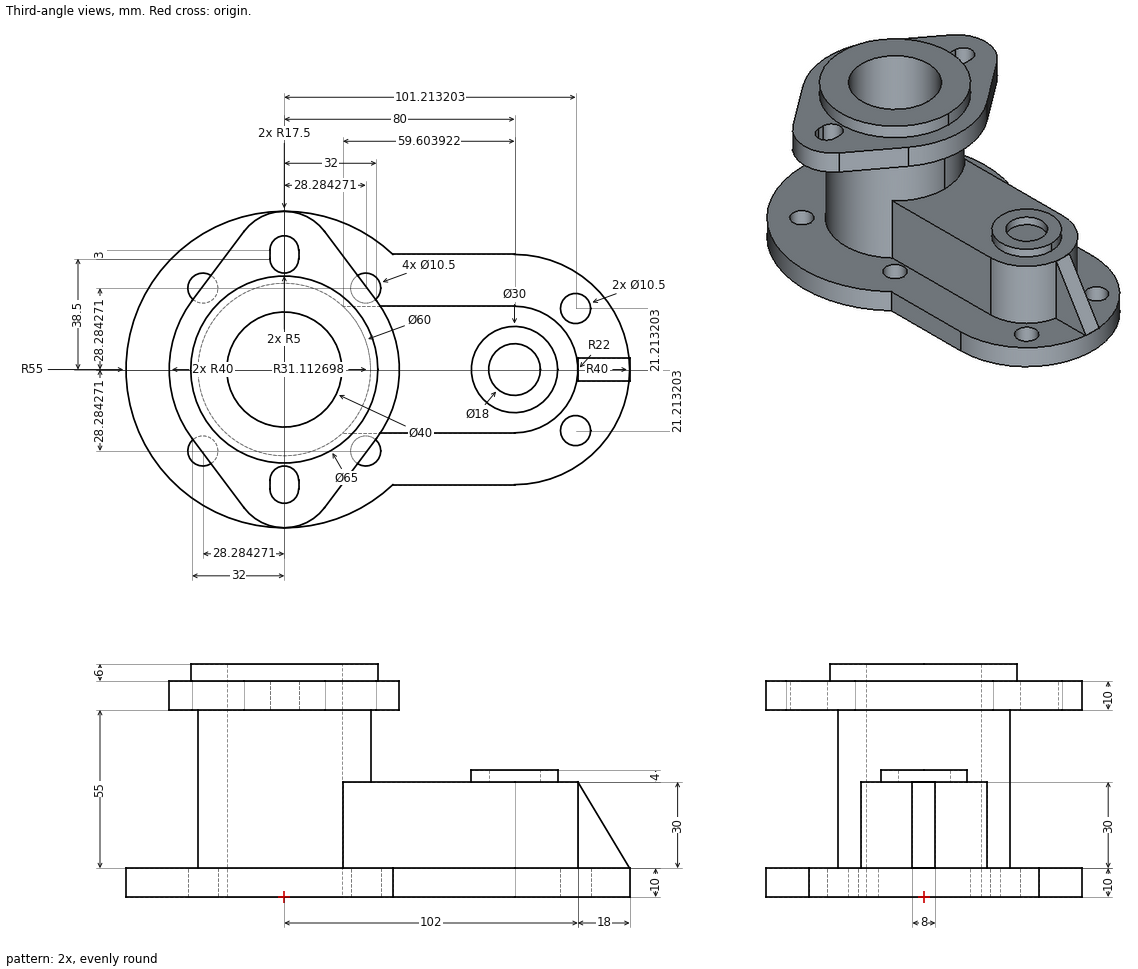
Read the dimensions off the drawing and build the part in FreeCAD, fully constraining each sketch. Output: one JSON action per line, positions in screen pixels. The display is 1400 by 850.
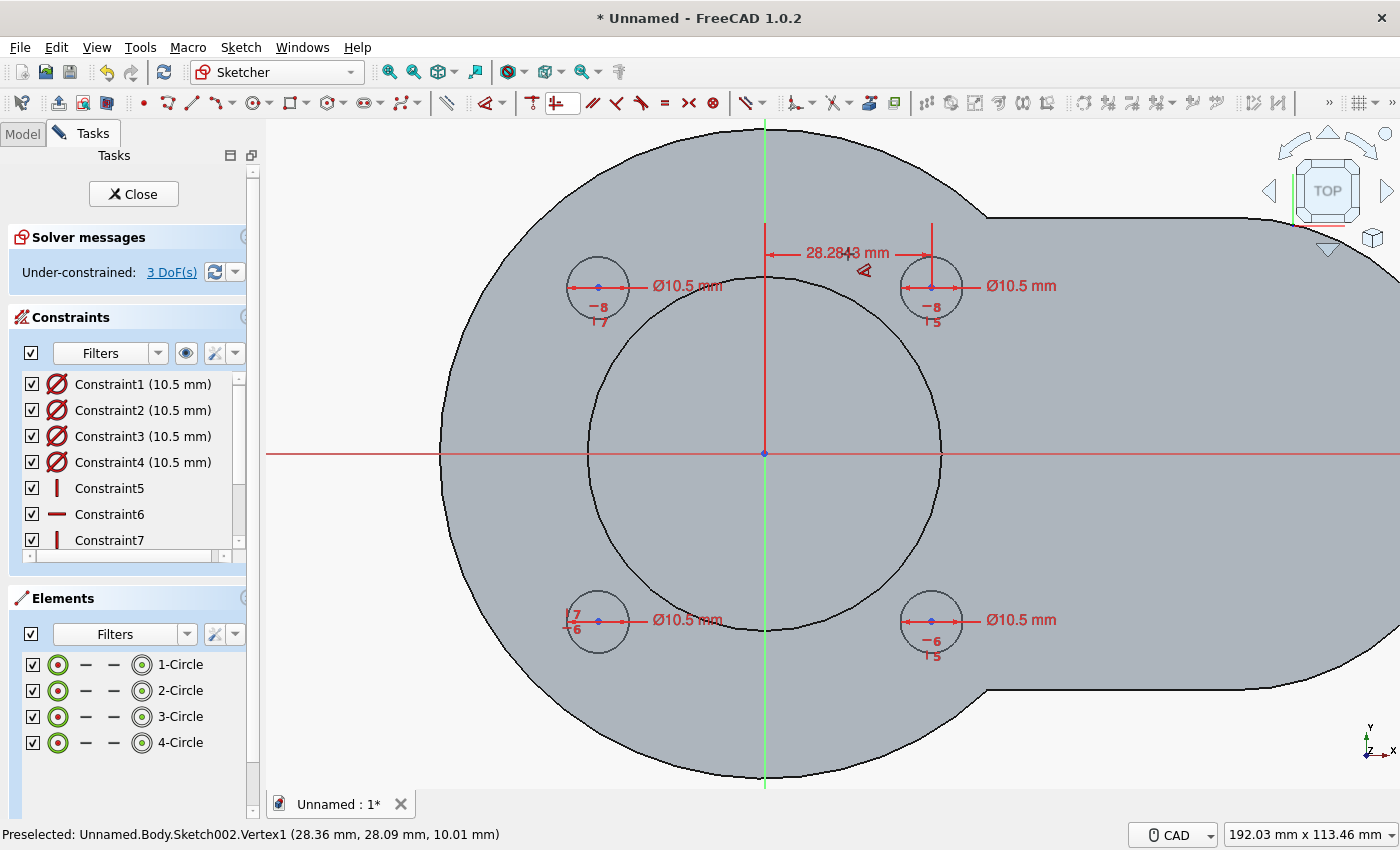
{"action": "left_click", "coordinate": [932, 288]}
{"action": "left_click", "coordinate": [966, 371]}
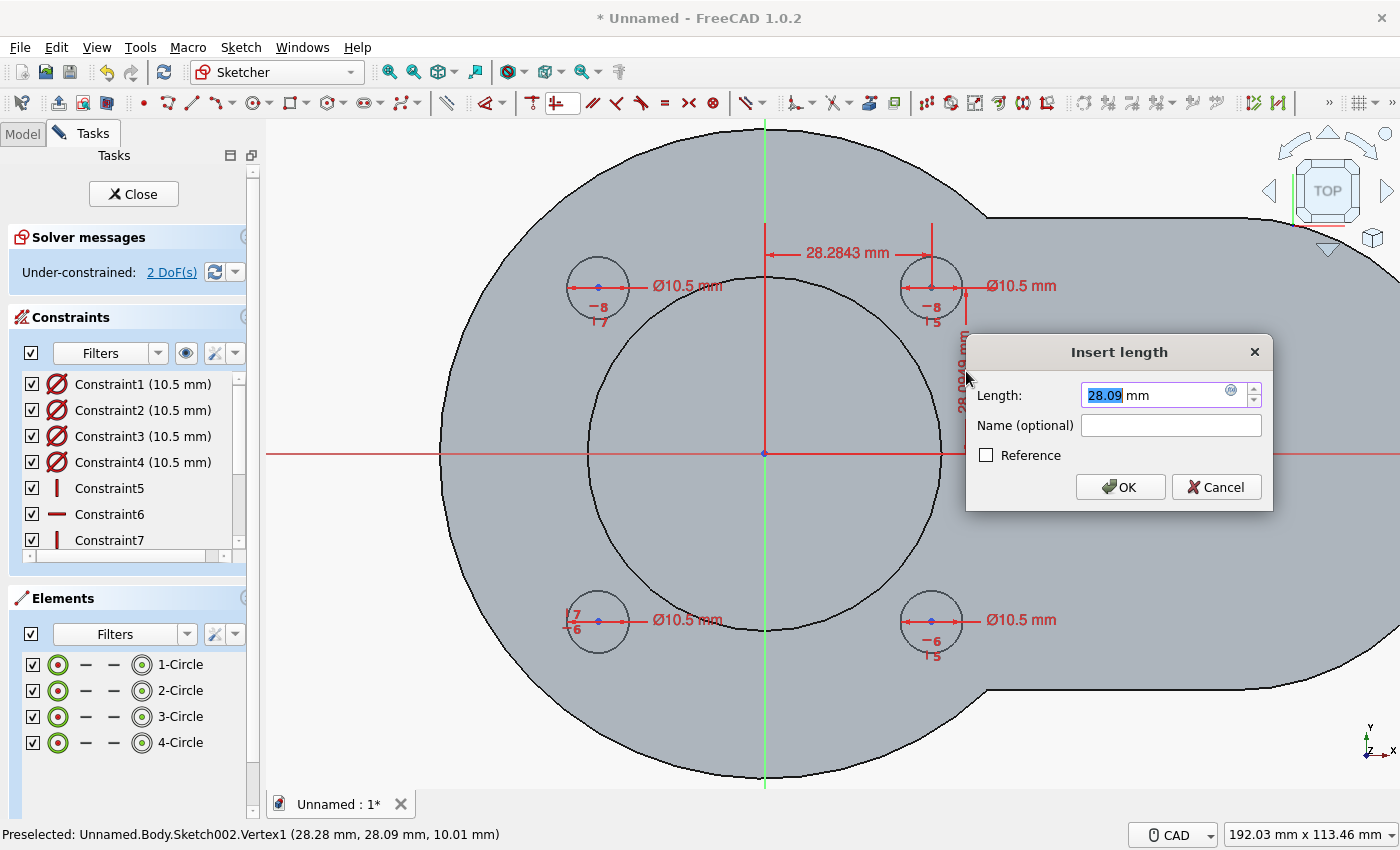
{"action": "type", "text": "28.284271"}
{"action": "key", "text": "Return"}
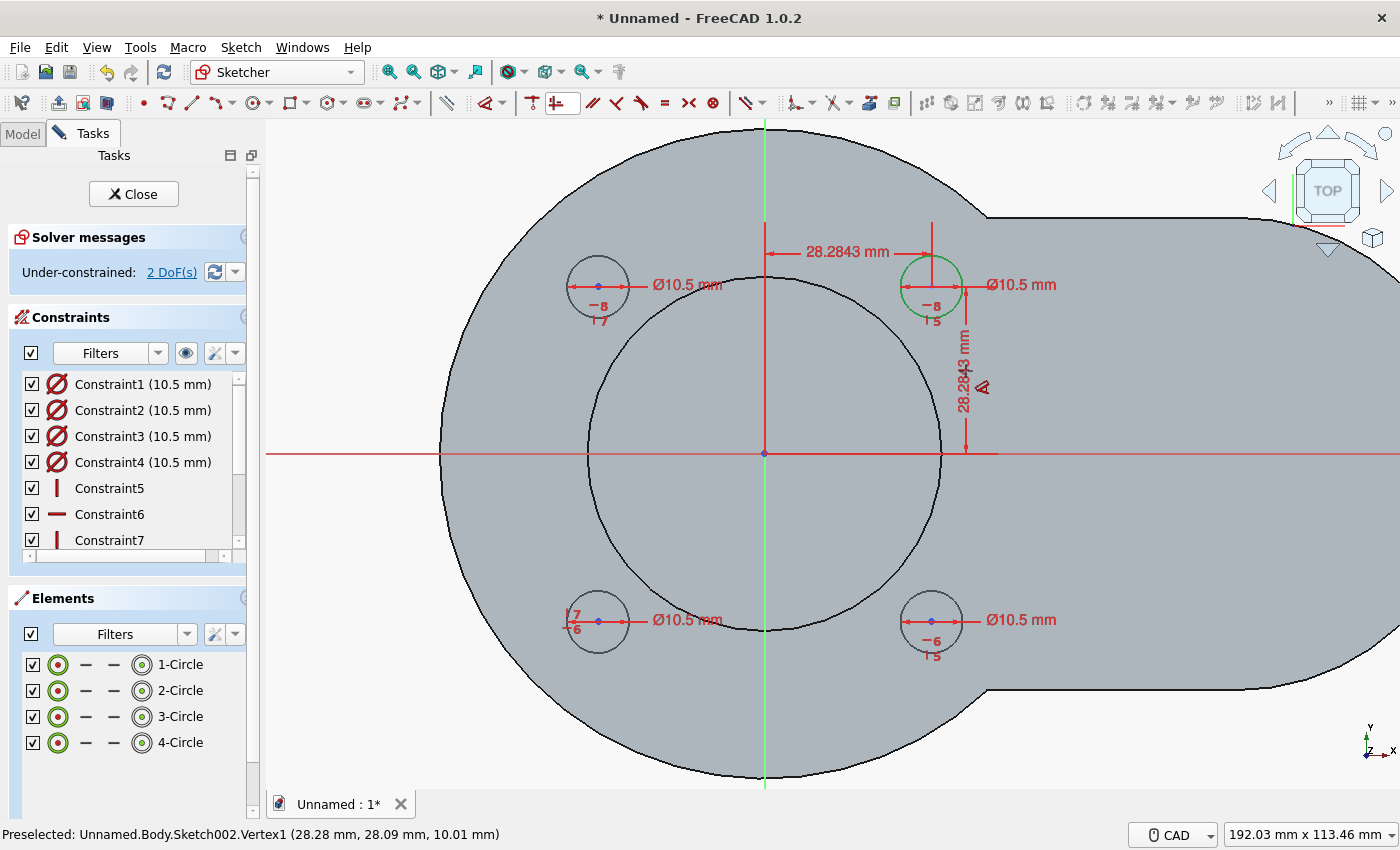
{"action": "left_click", "coordinate": [932, 622]}
{"action": "left_click", "coordinate": [966, 538]}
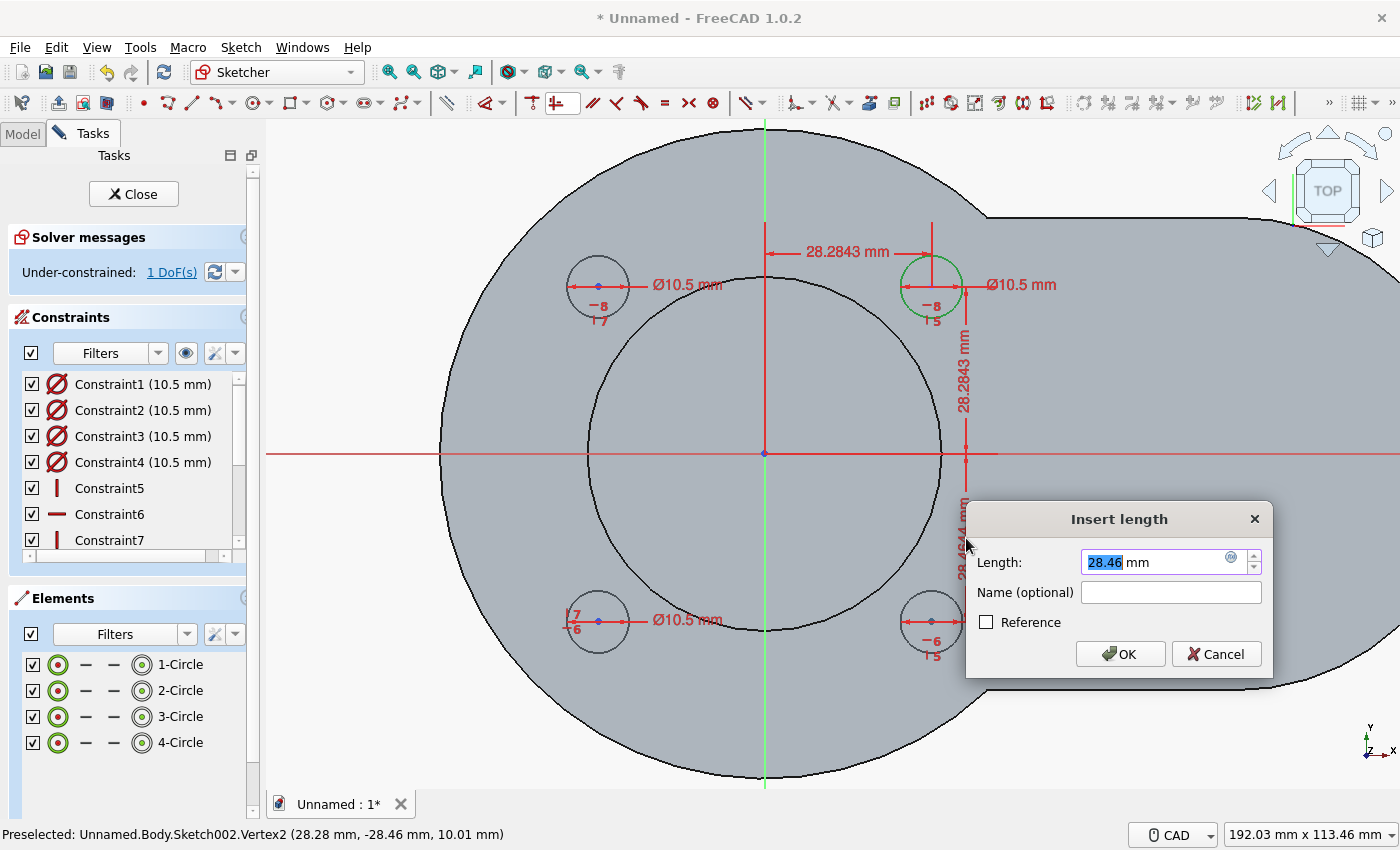
{"action": "type", "text": "28.284271"}
{"action": "key", "text": "Return"}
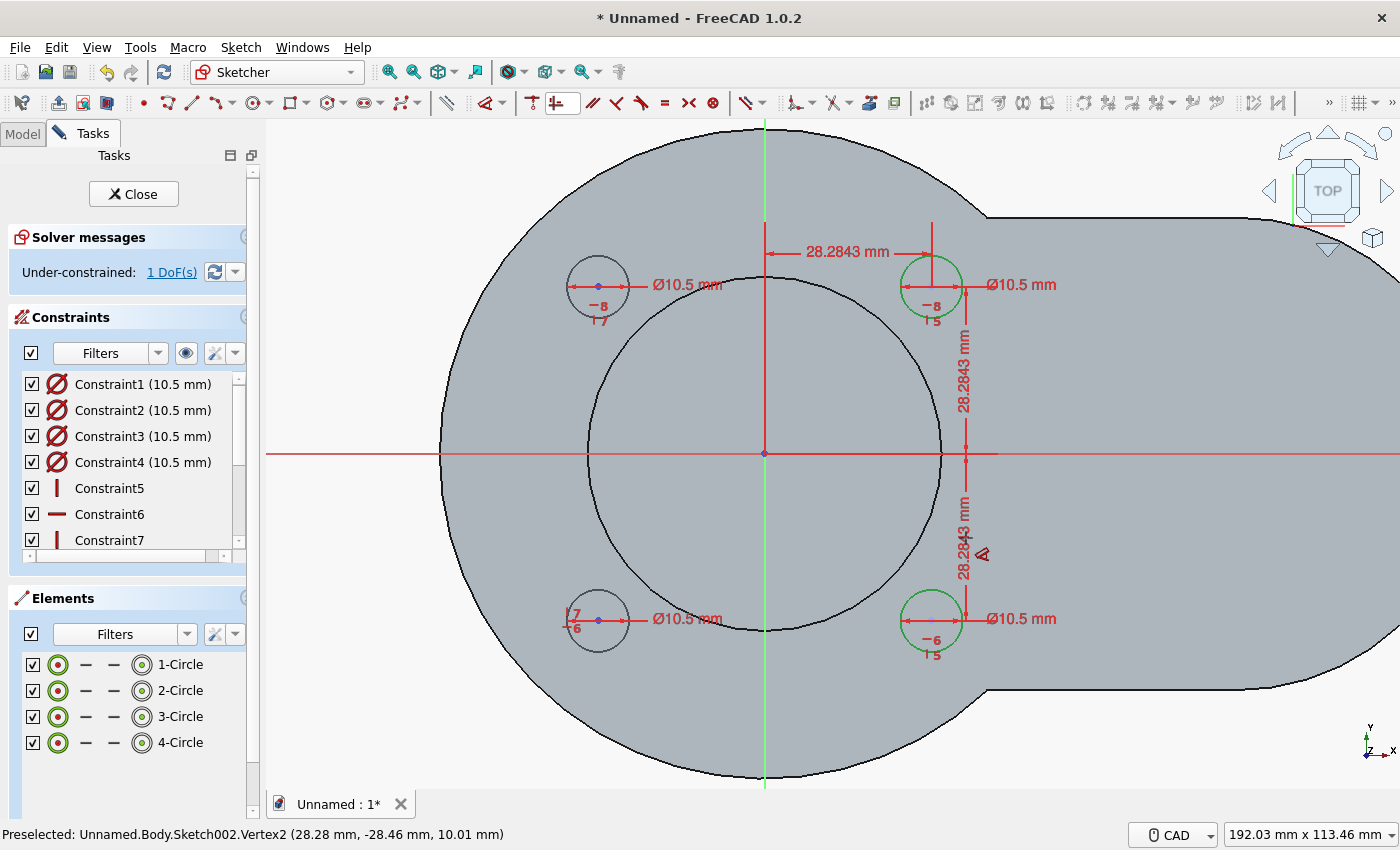
{"action": "left_click", "coordinate": [598, 621]}
{"action": "left_click", "coordinate": [681, 655]}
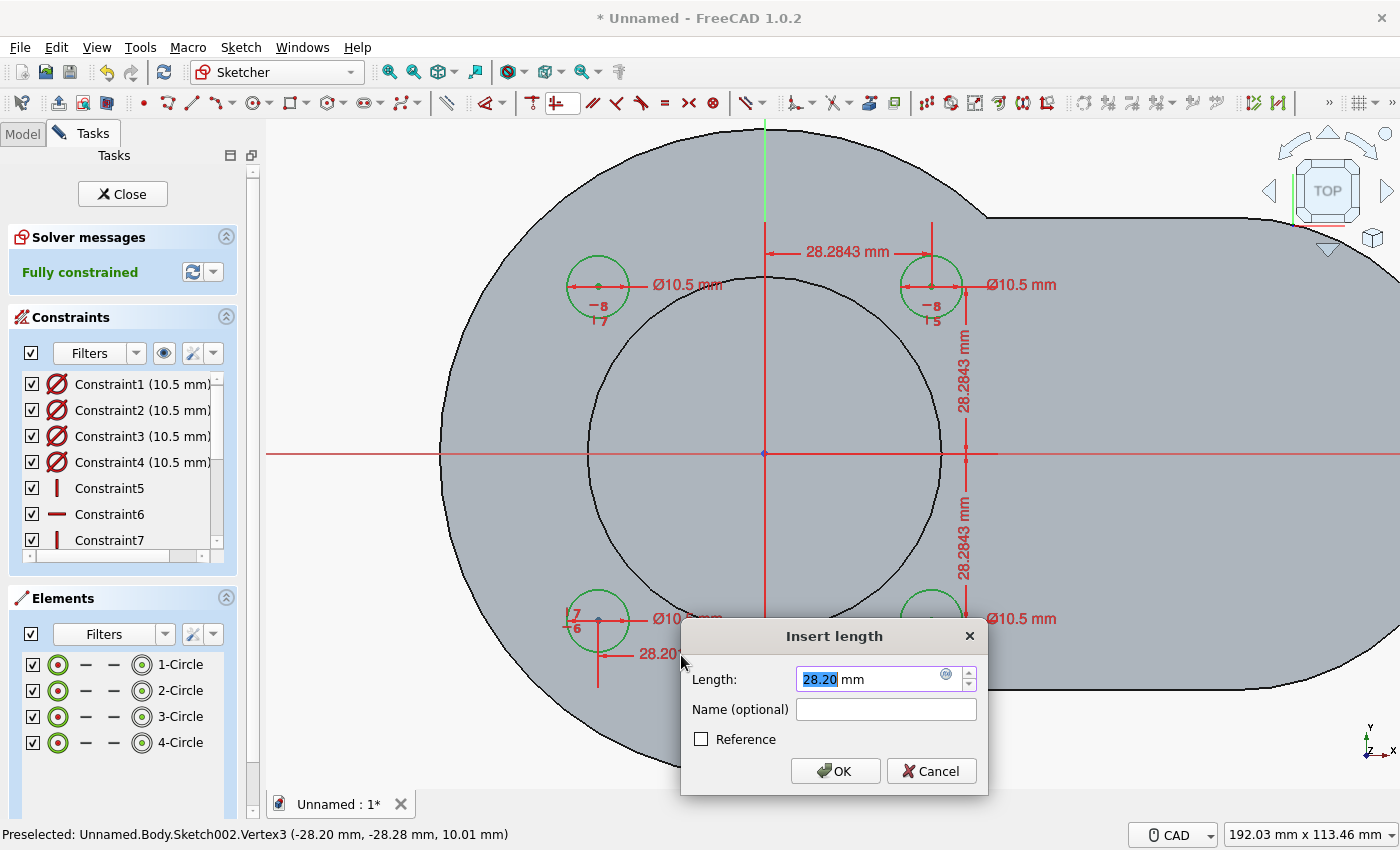
{"action": "type", "text": "28.284271"}
{"action": "key", "text": "Return"}
{"action": "key", "text": "Escape"}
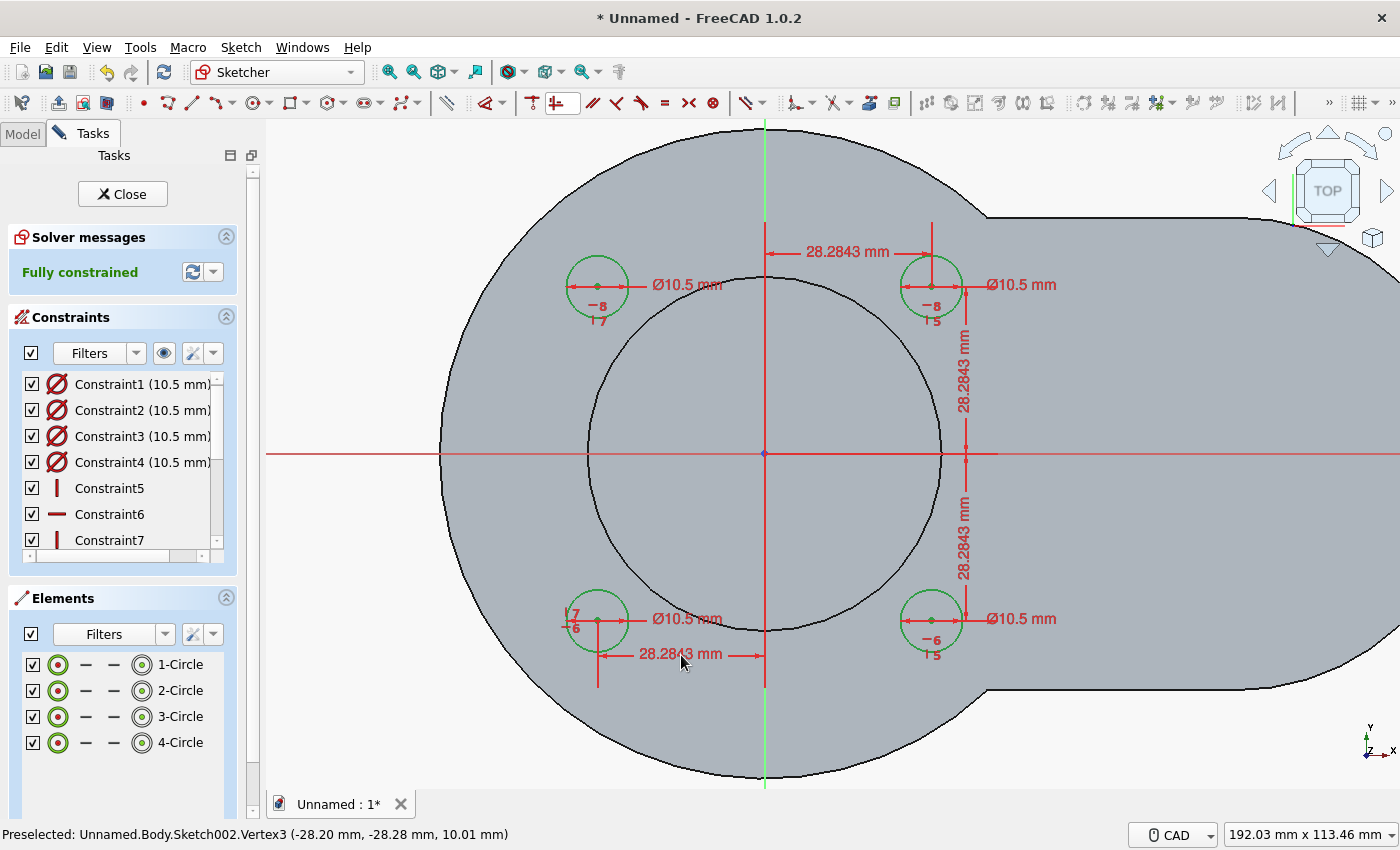
{"action": "left_click", "coordinate": [123, 194]}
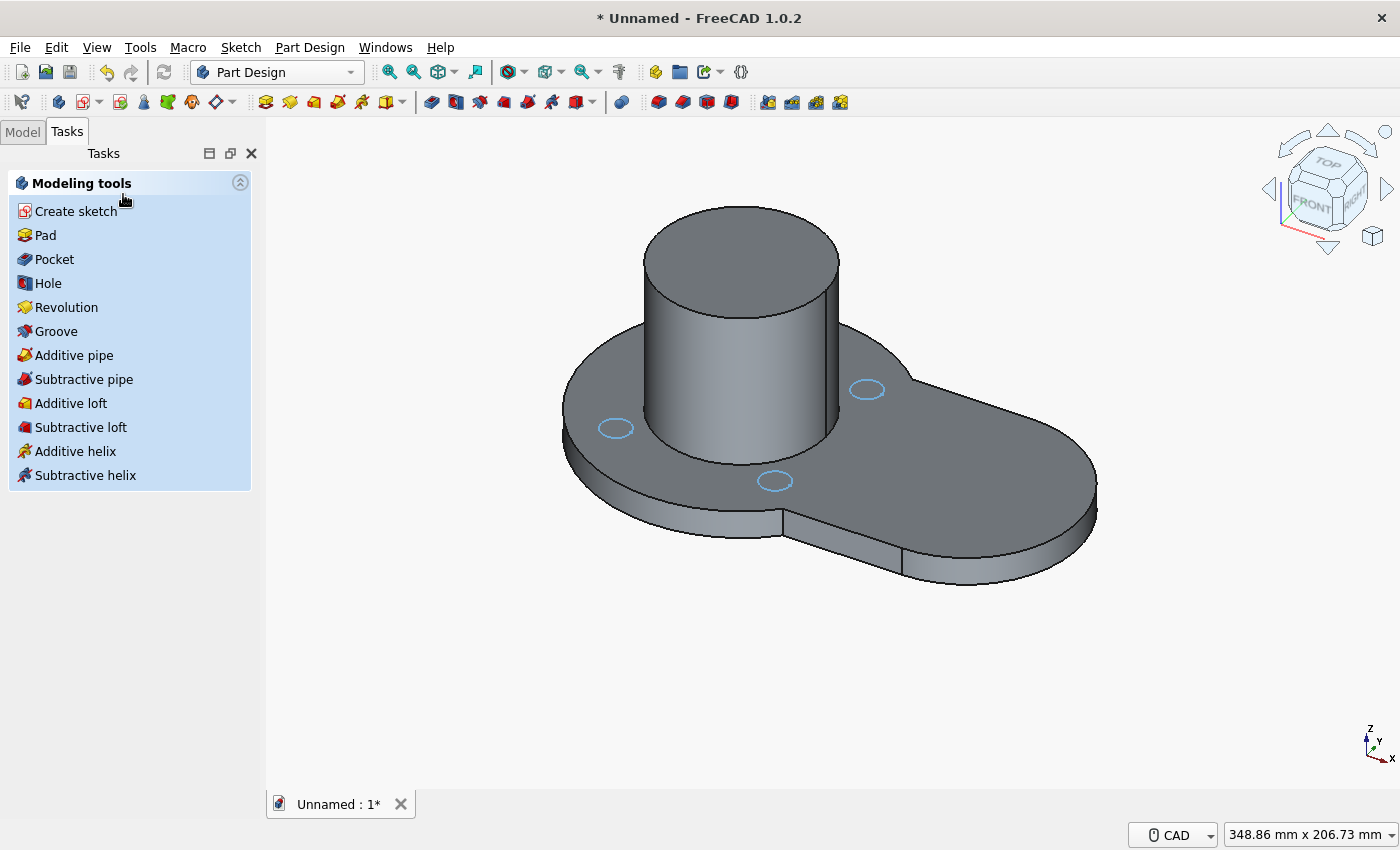
{"action": "left_click", "coordinate": [432, 102]}